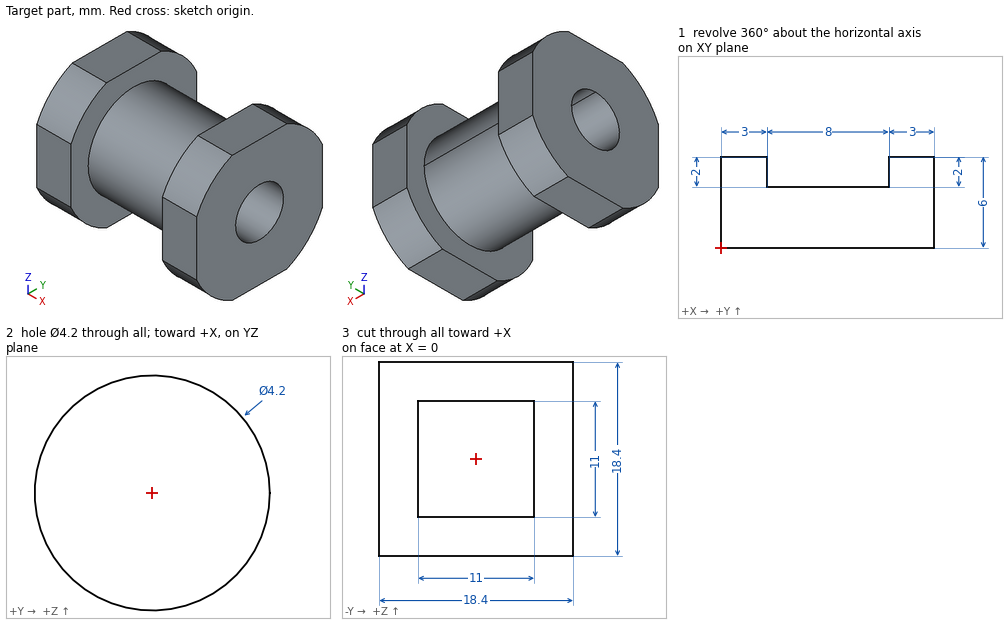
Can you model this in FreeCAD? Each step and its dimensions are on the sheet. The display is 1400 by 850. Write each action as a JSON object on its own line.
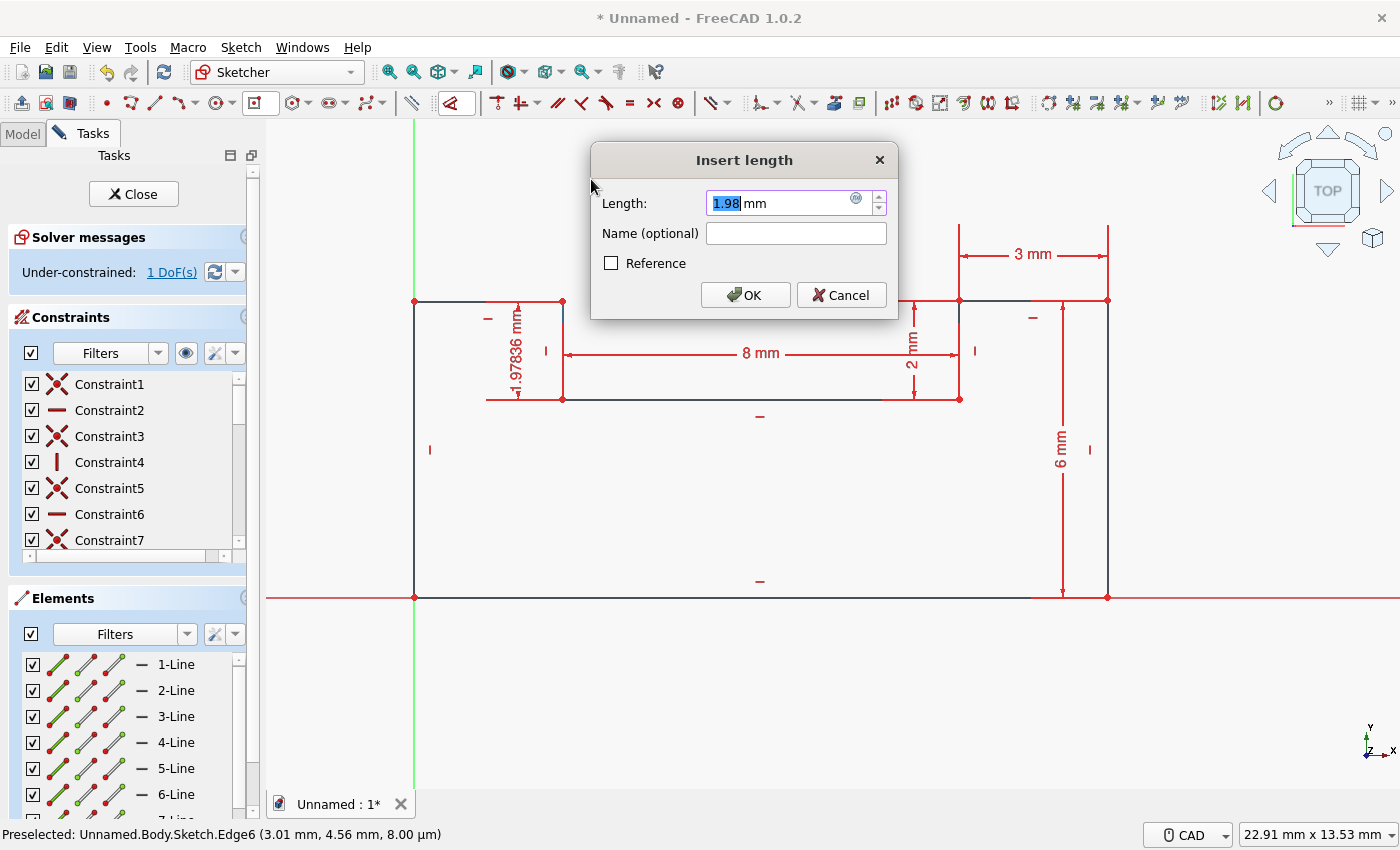
{"action": "type", "text": "2"}
{"action": "key", "text": "Return"}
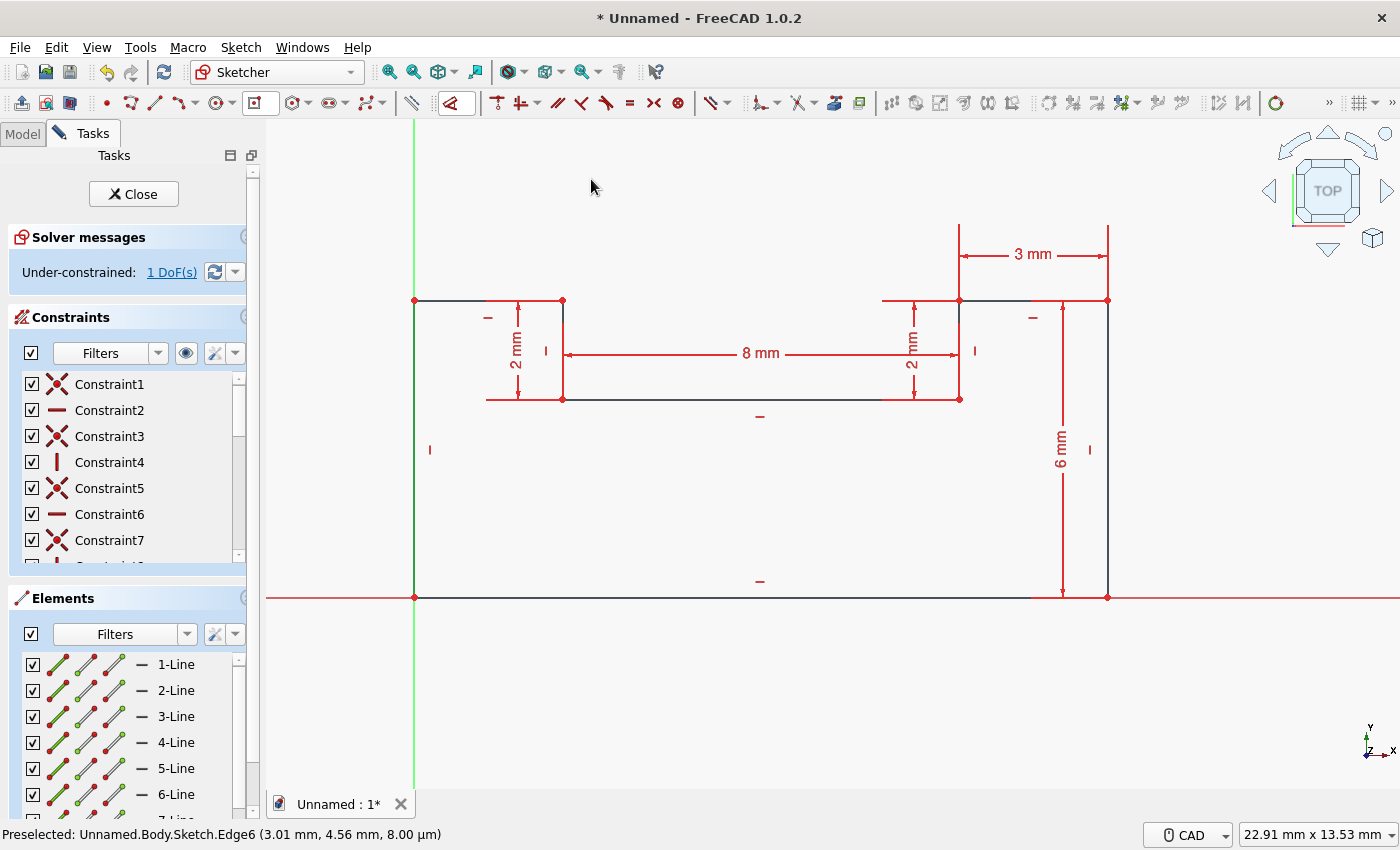
{"action": "left_click", "coordinate": [518, 301]}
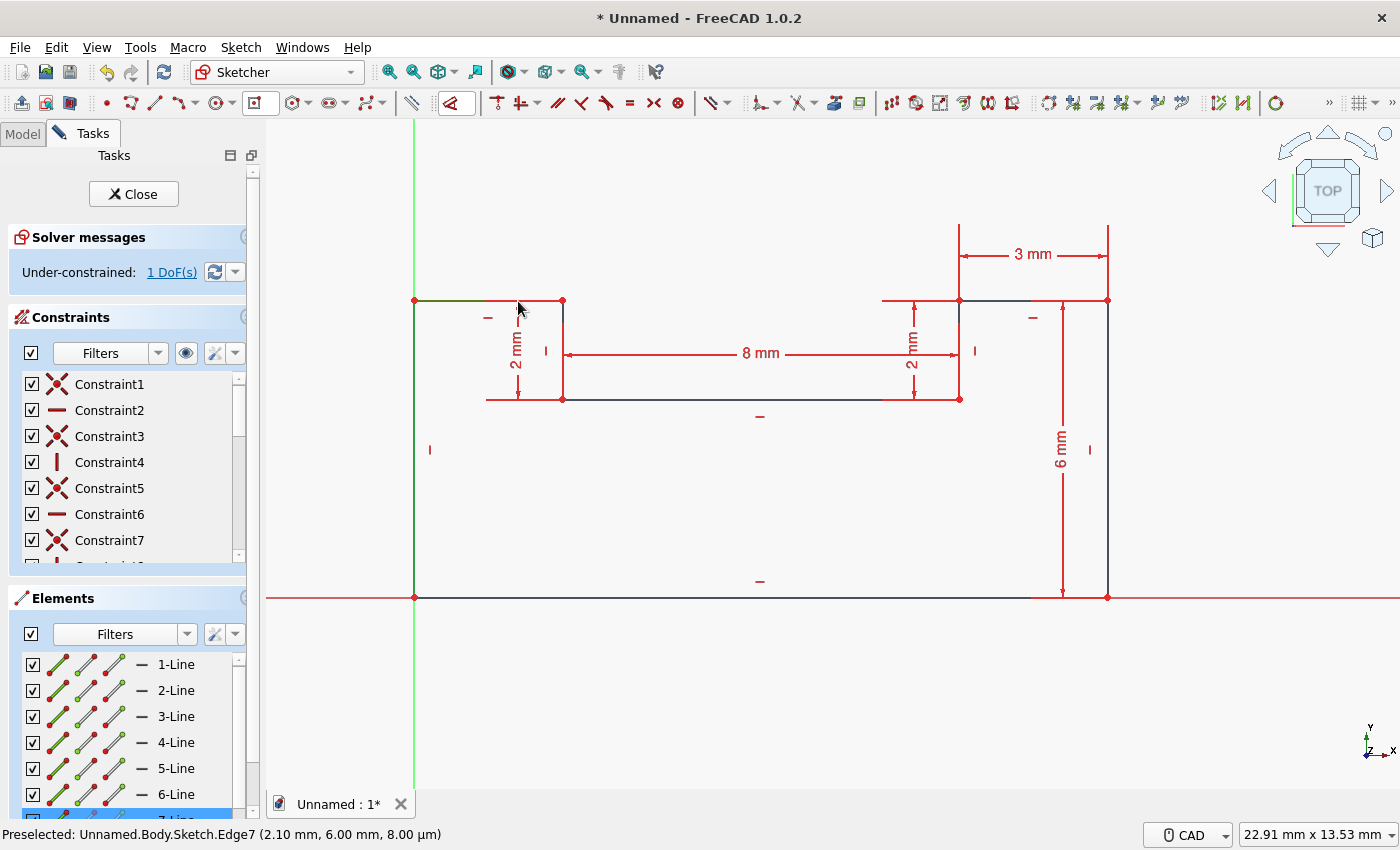
{"action": "left_click", "coordinate": [470, 104]}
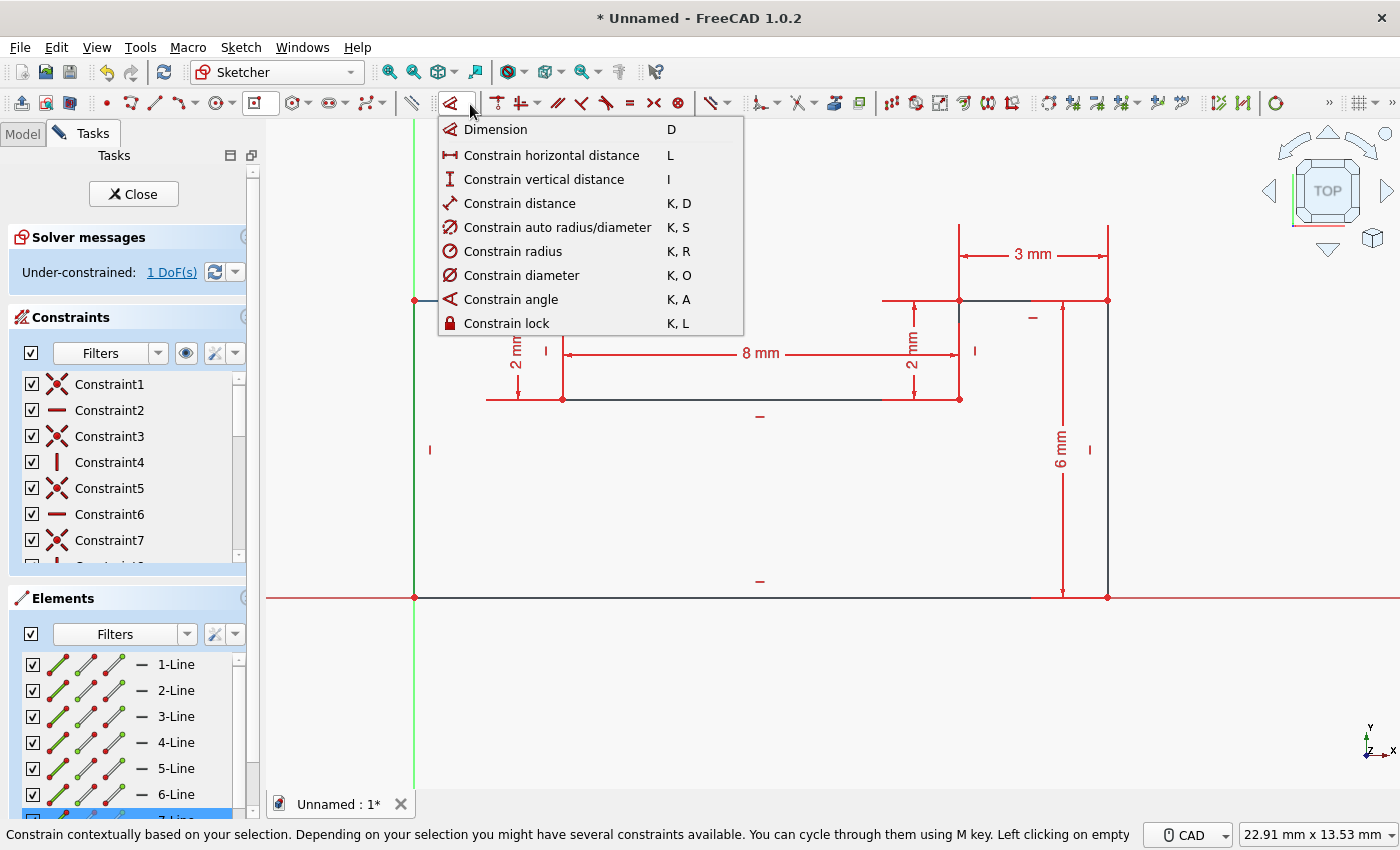
{"action": "left_click", "coordinate": [591, 155]}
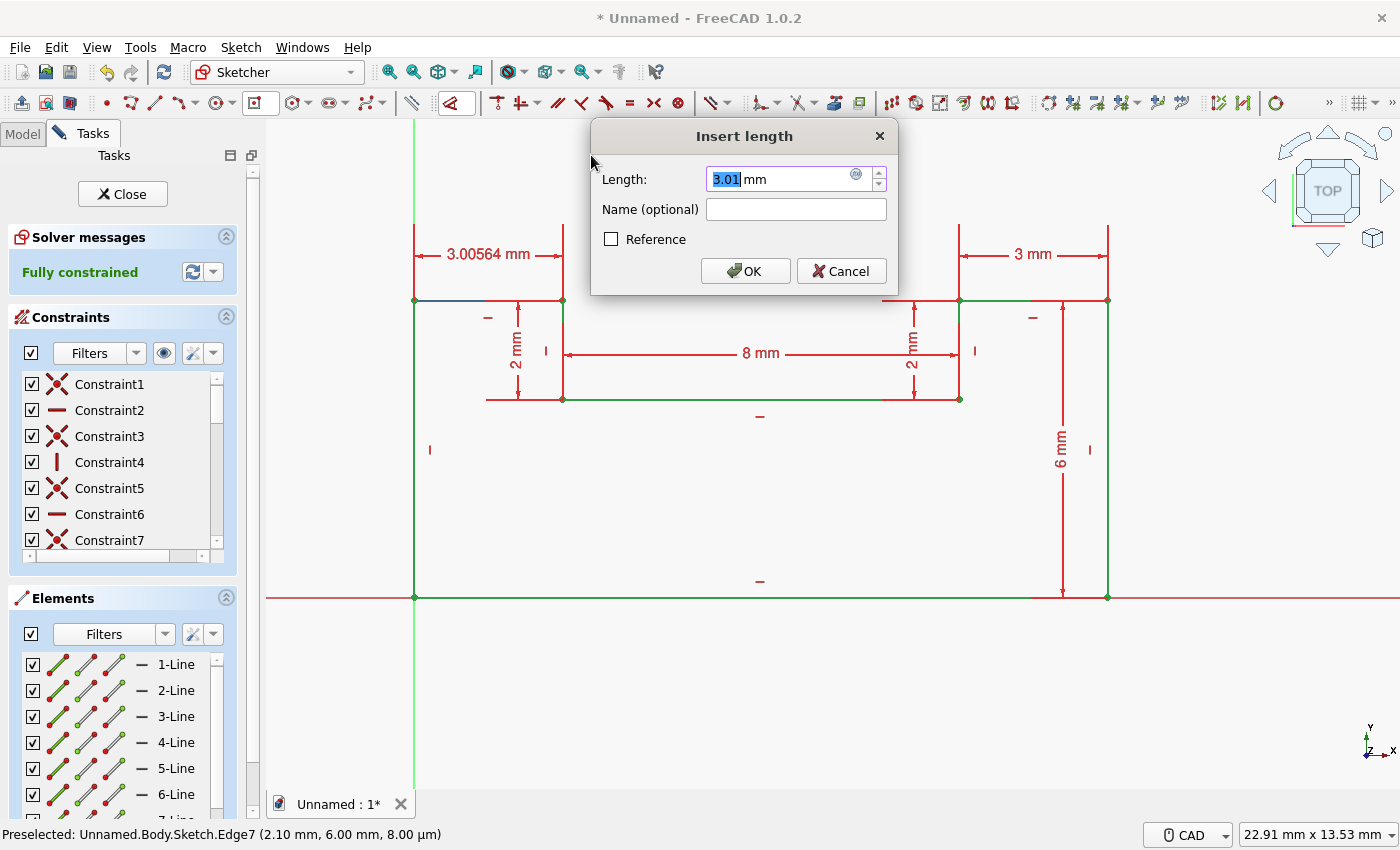
{"action": "type", "text": "3"}
{"action": "key", "text": "Return"}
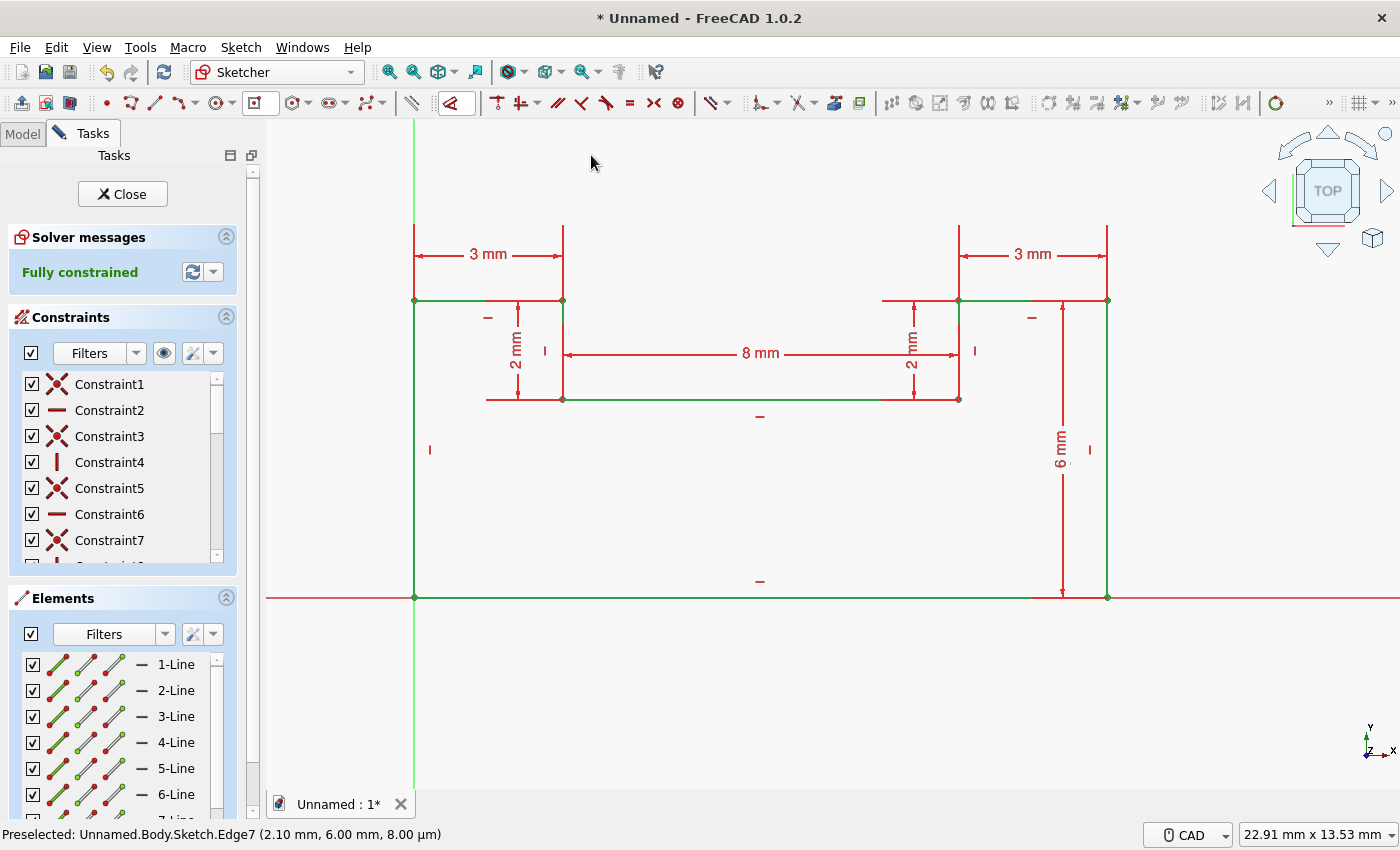
{"action": "left_click", "coordinate": [123, 194]}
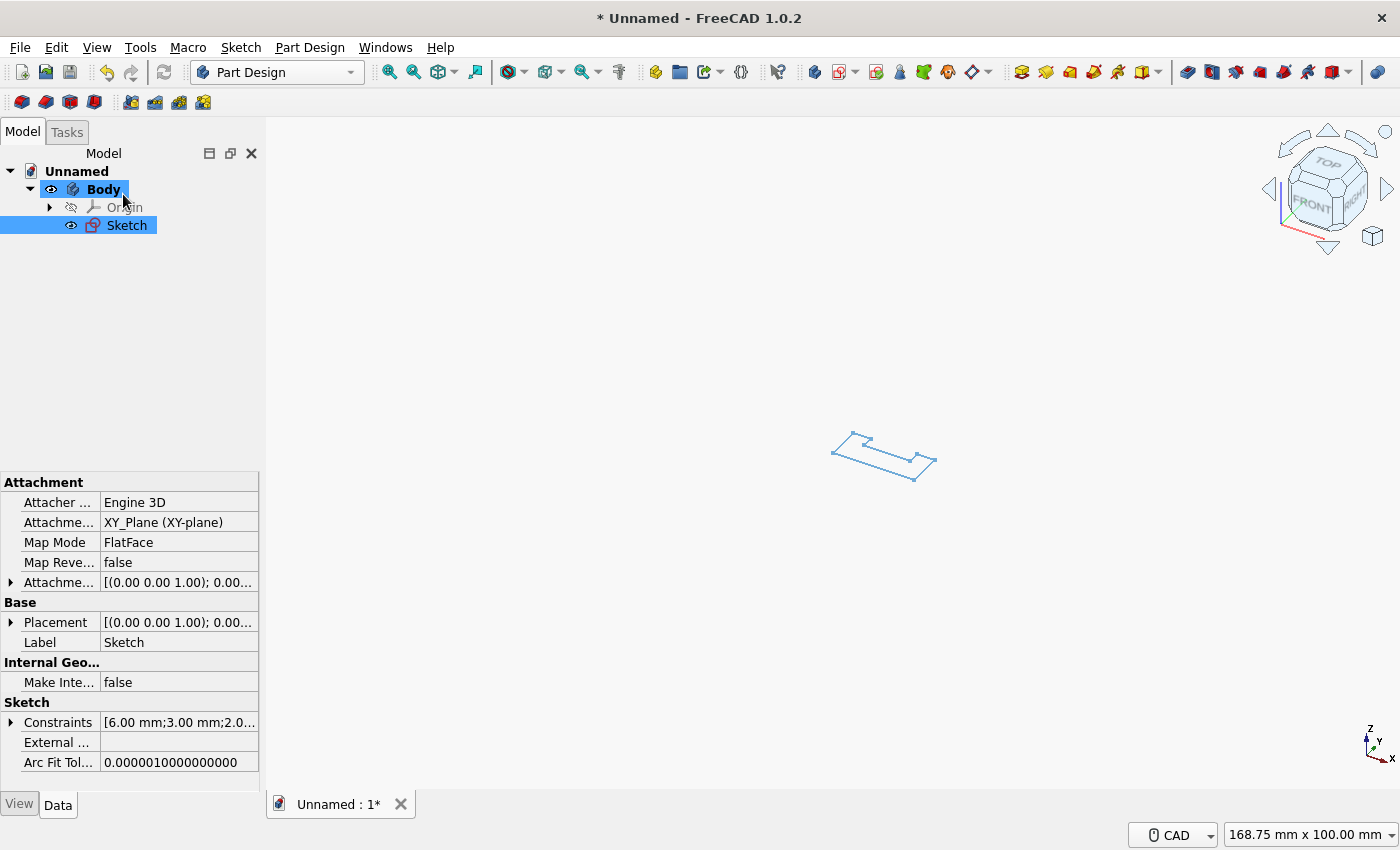
{"action": "left_click", "coordinate": [1046, 72]}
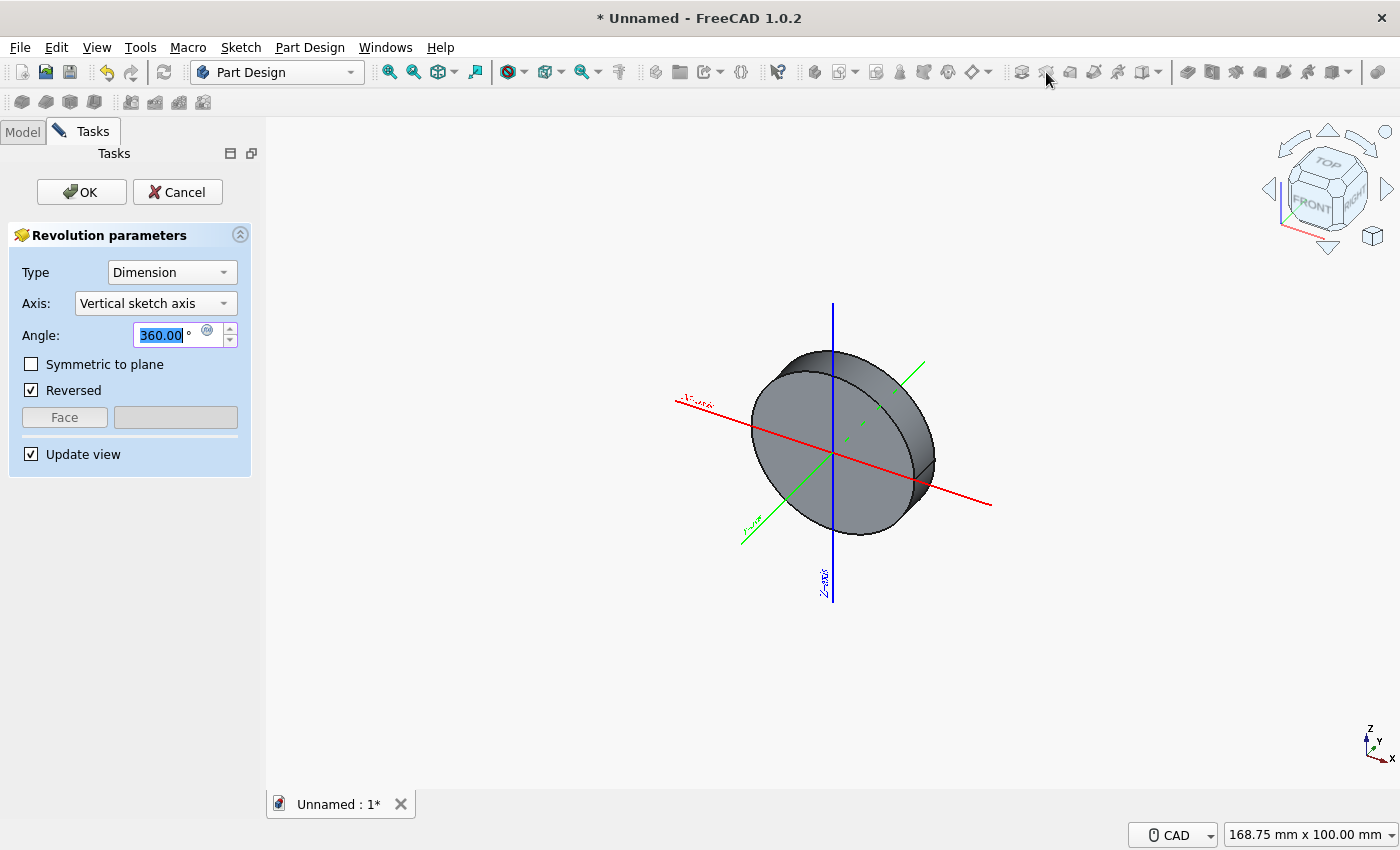
{"action": "left_click", "coordinate": [156, 304]}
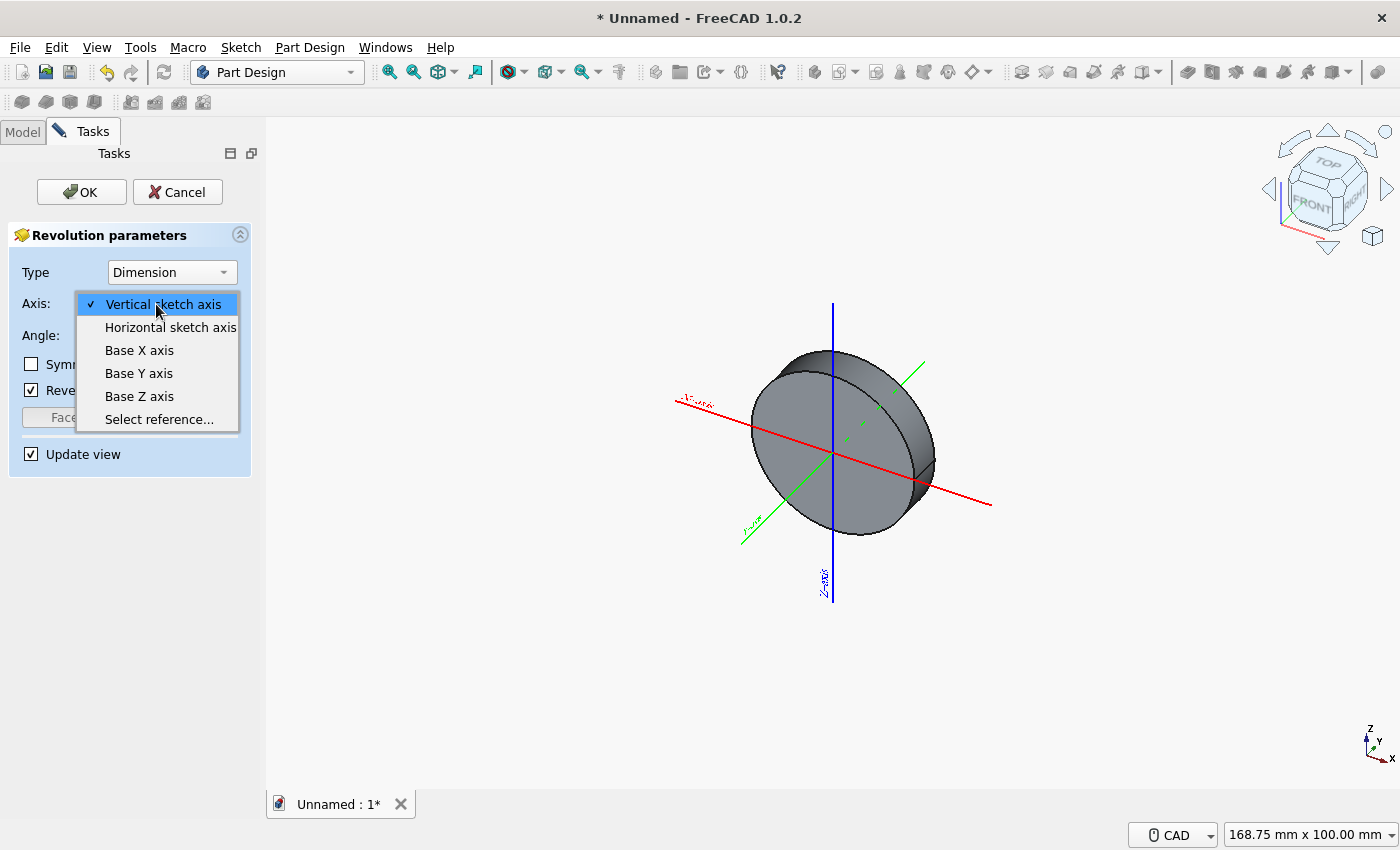
{"action": "left_click", "coordinate": [156, 328]}